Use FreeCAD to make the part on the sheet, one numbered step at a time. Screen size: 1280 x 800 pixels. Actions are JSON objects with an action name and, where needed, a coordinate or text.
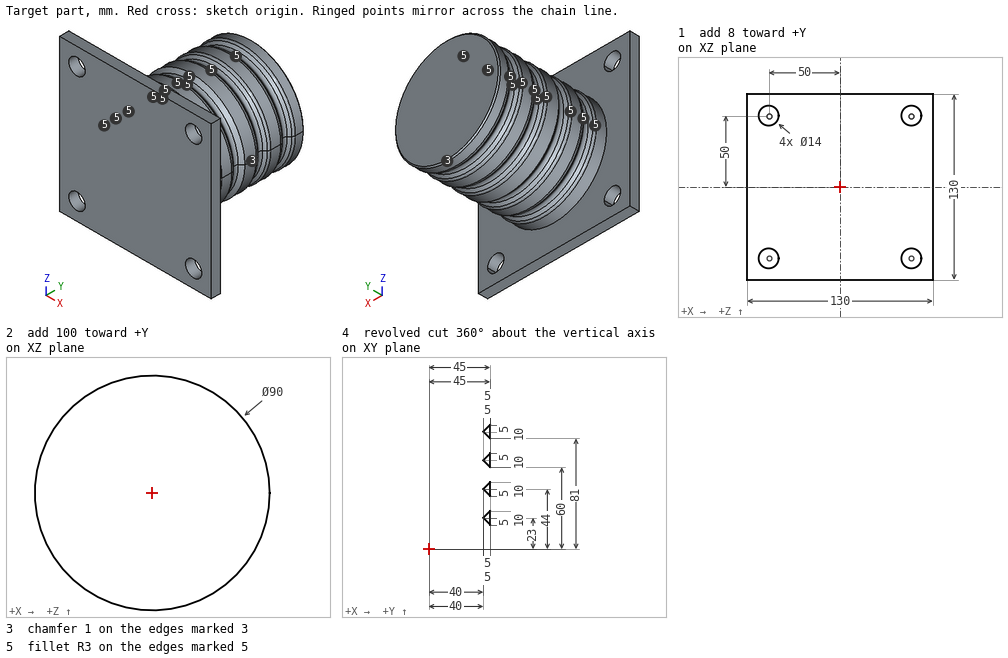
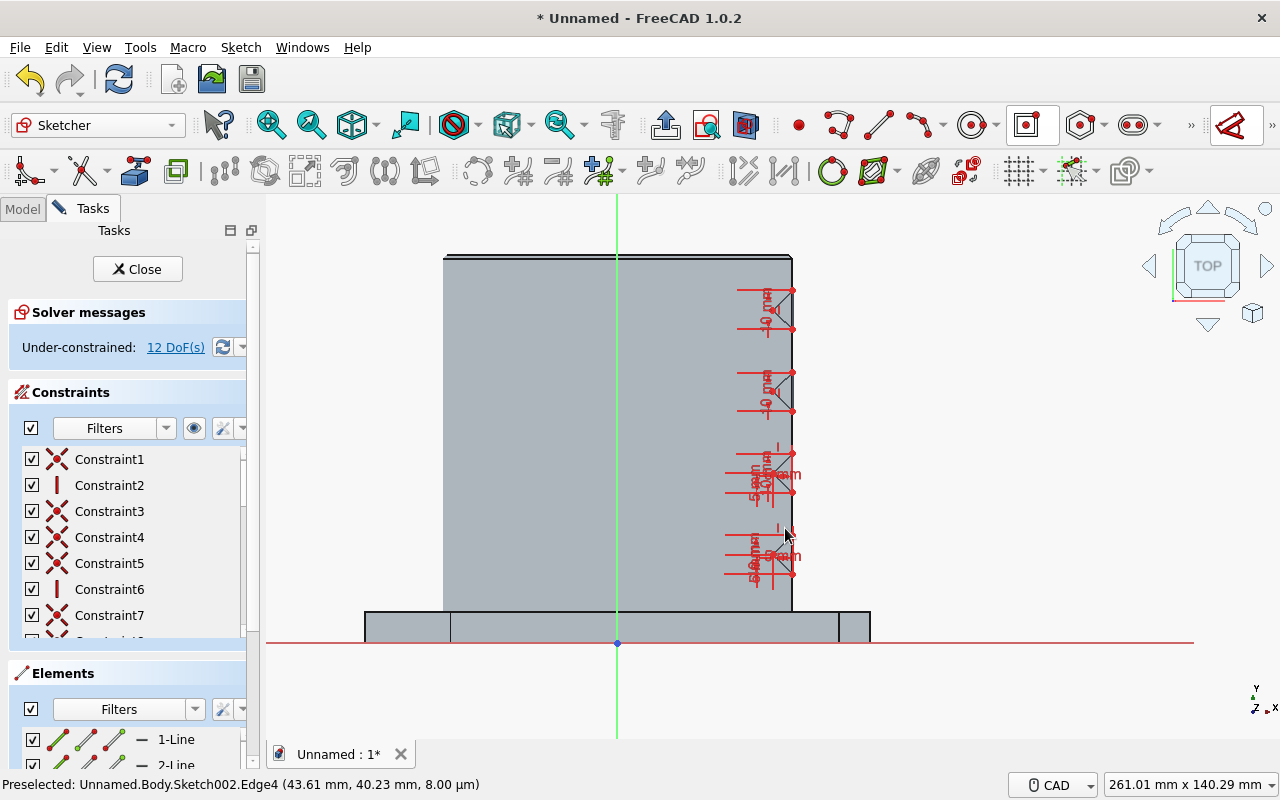
{"action": "scroll", "coordinate": [787, 378], "scroll_direction": "up", "scroll_amount": 5}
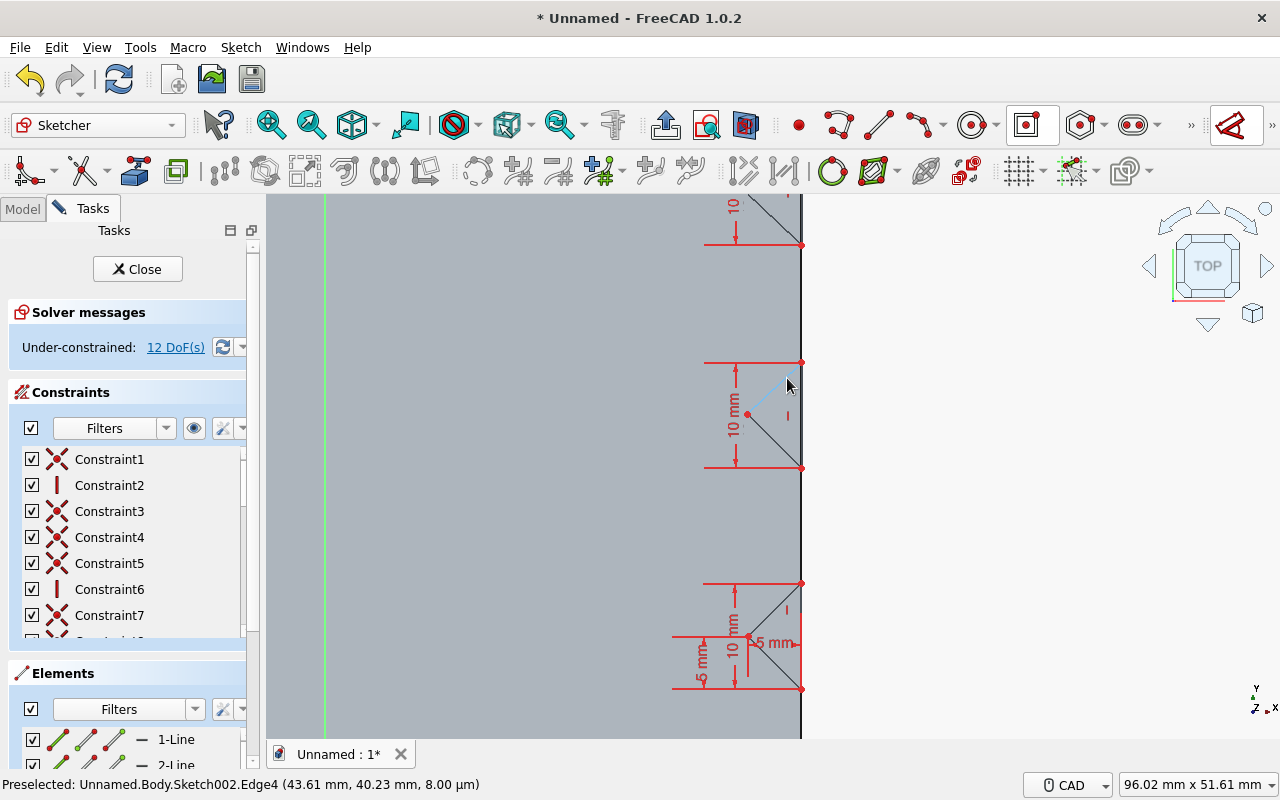
{"action": "left_click", "coordinate": [786, 378]}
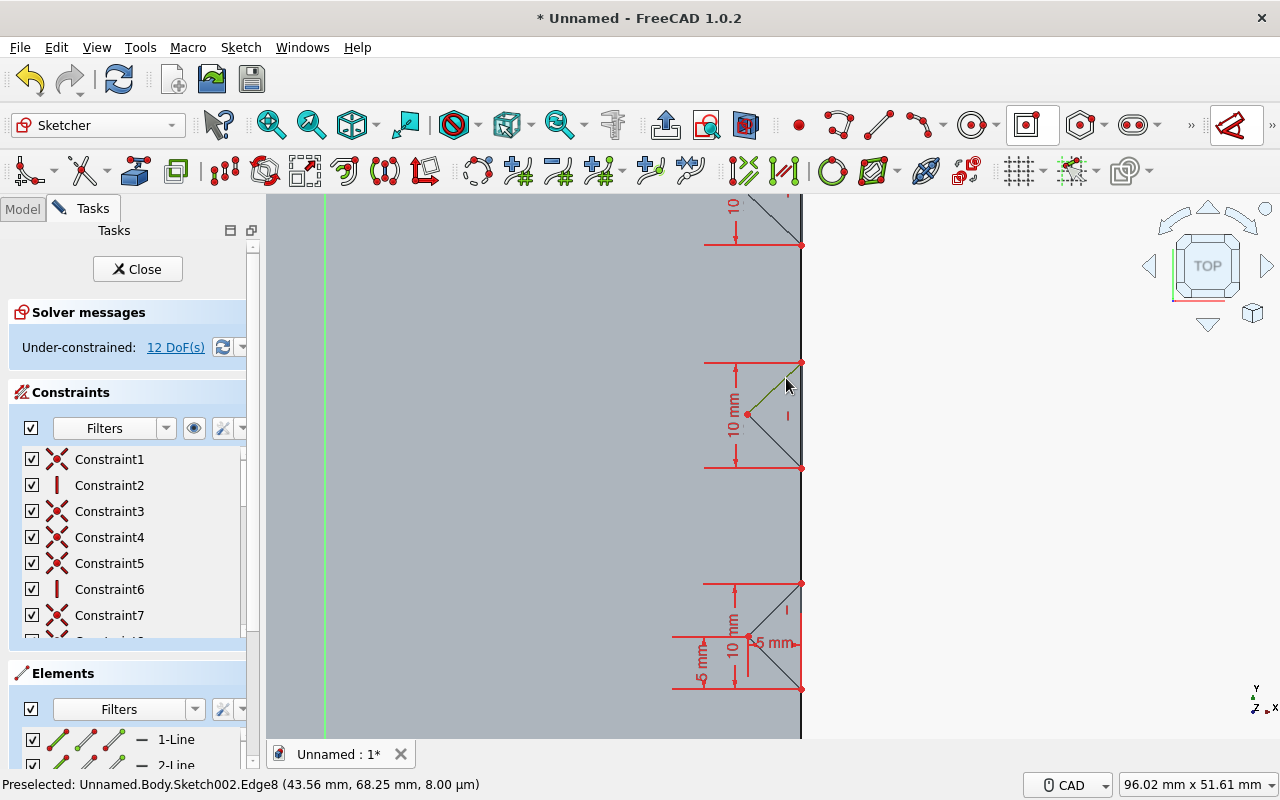
{"action": "left_click", "coordinate": [1258, 126]}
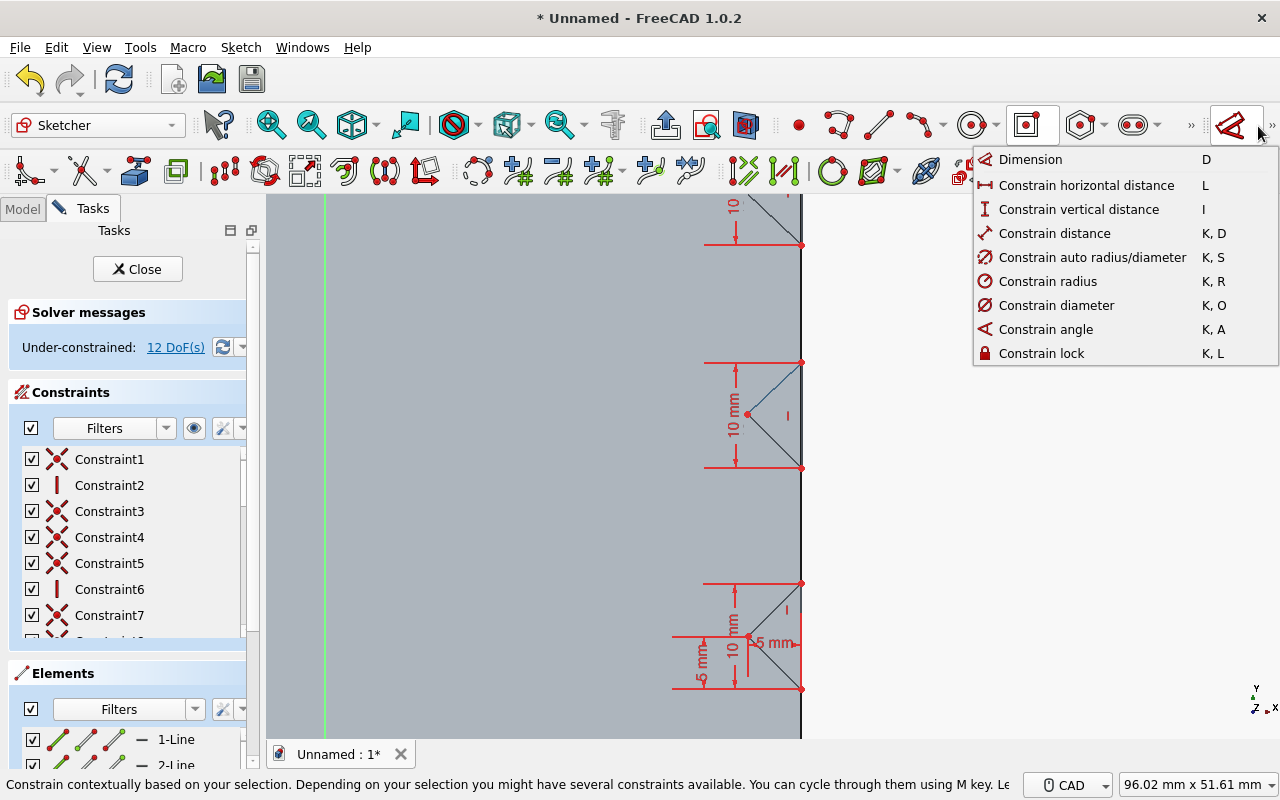
{"action": "left_click", "coordinate": [1126, 185]}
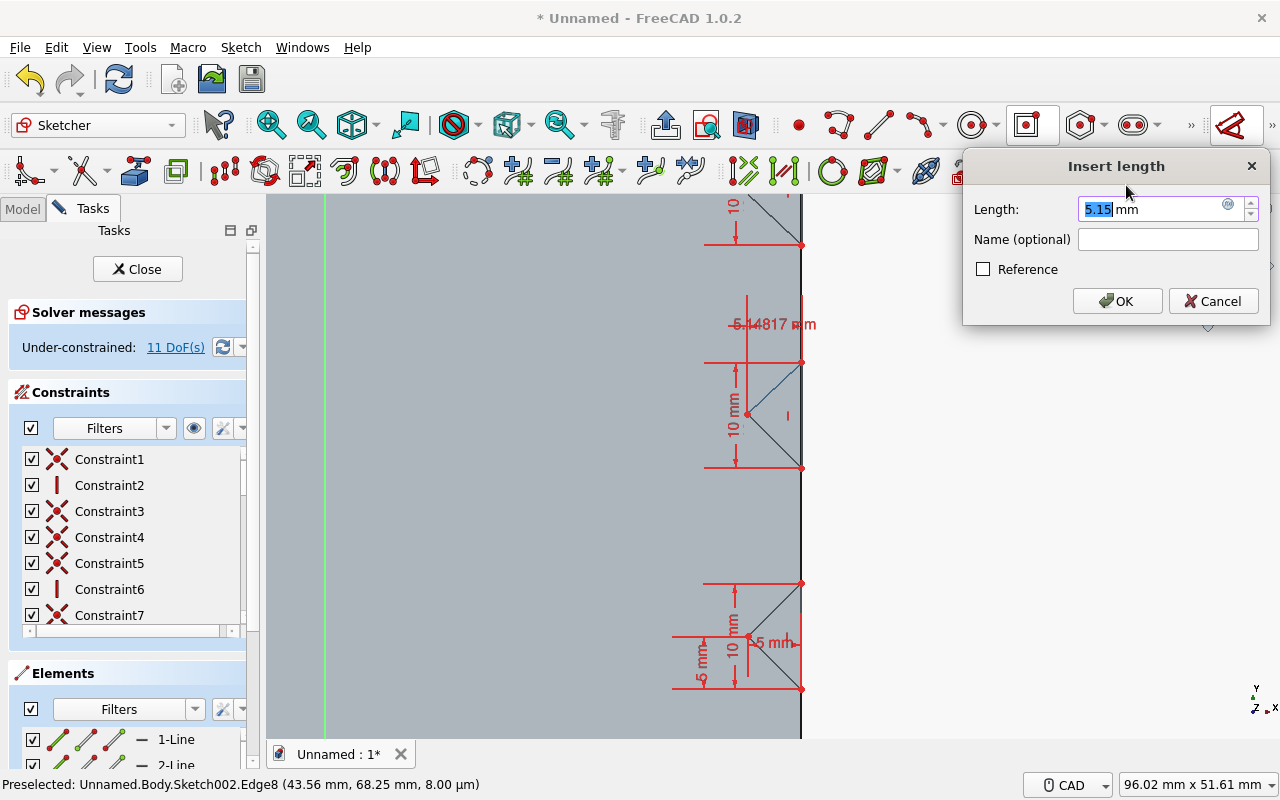
{"action": "type", "text": "5"}
{"action": "key", "text": "Return"}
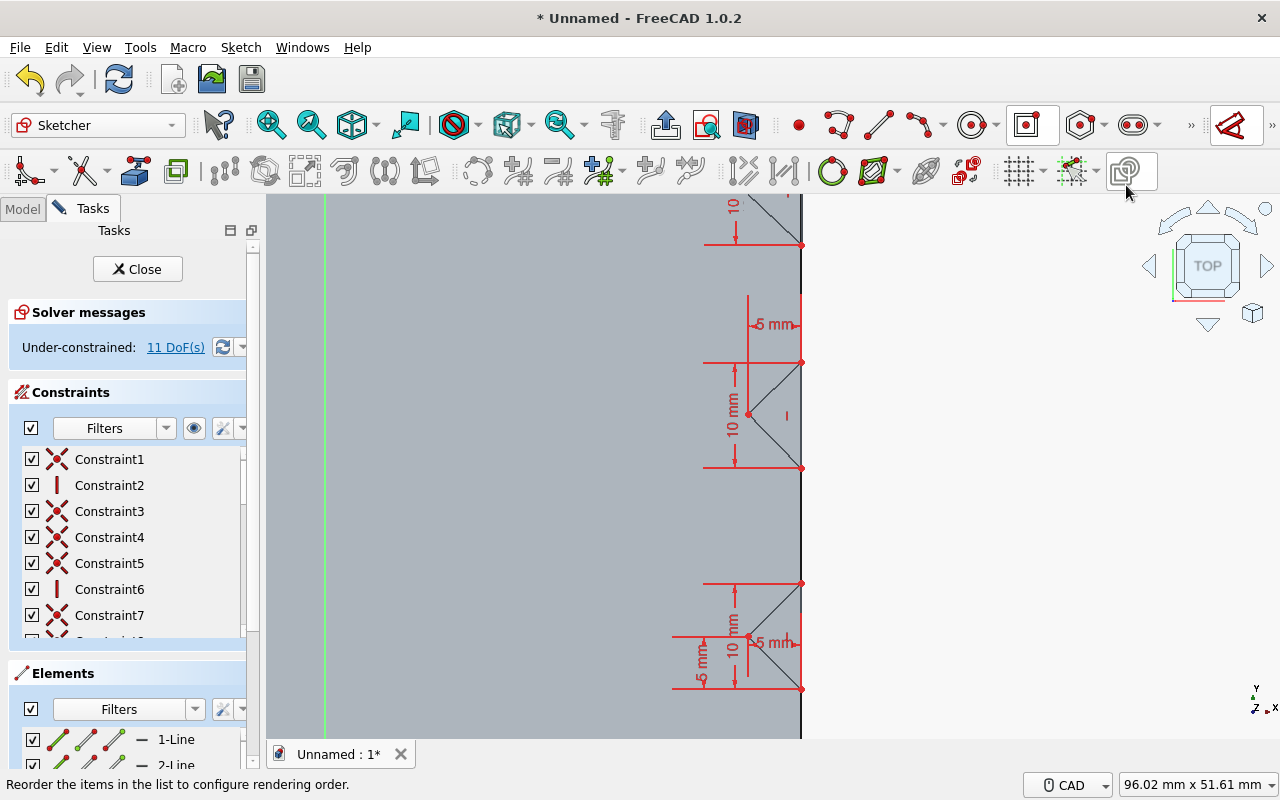
{"action": "left_click", "coordinate": [785, 378]}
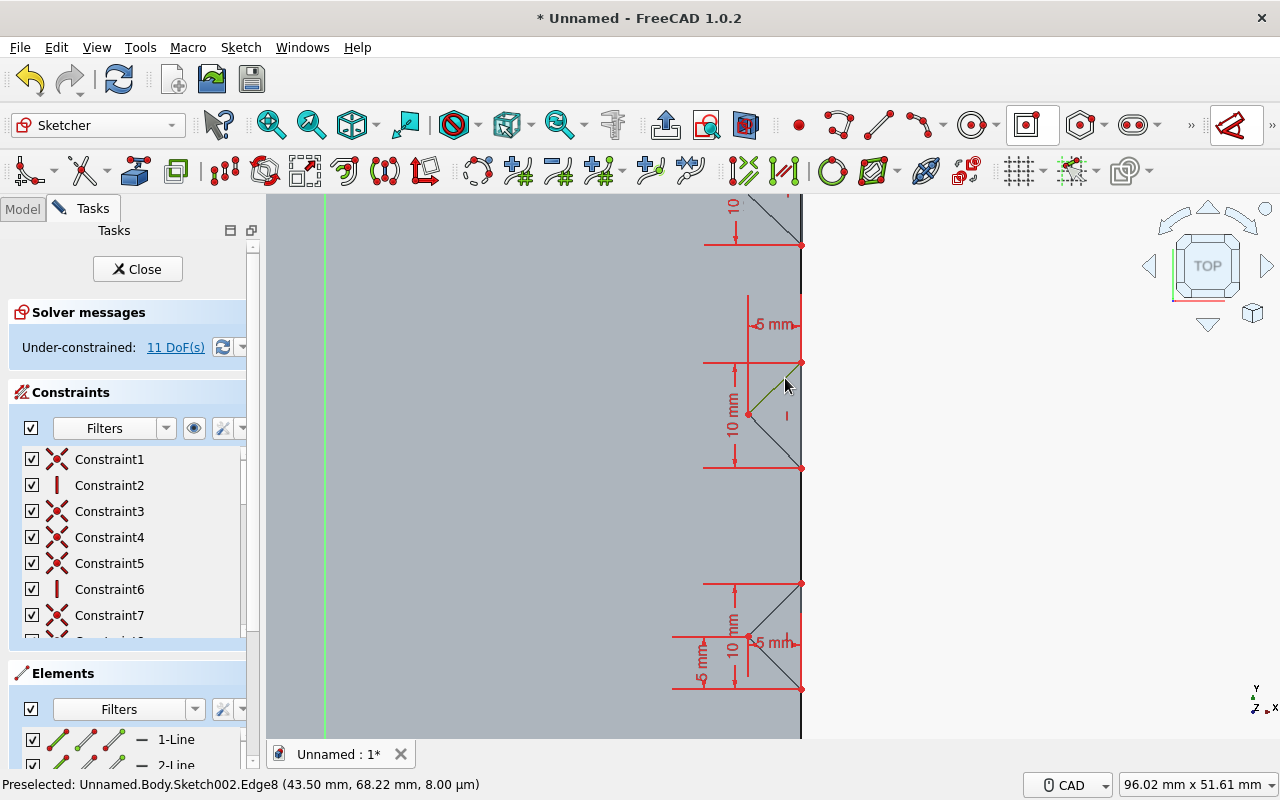
{"action": "left_click", "coordinate": [1258, 126]}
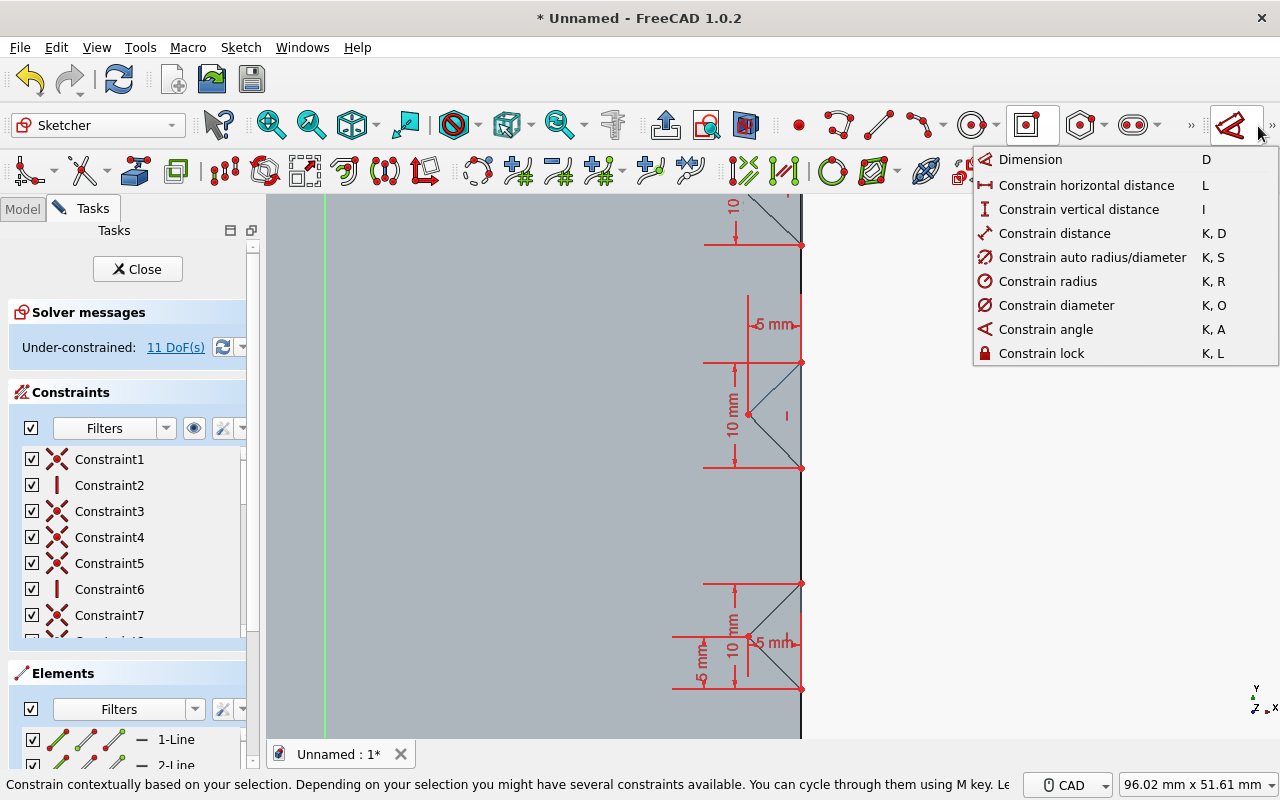
{"action": "left_click", "coordinate": [1126, 209]}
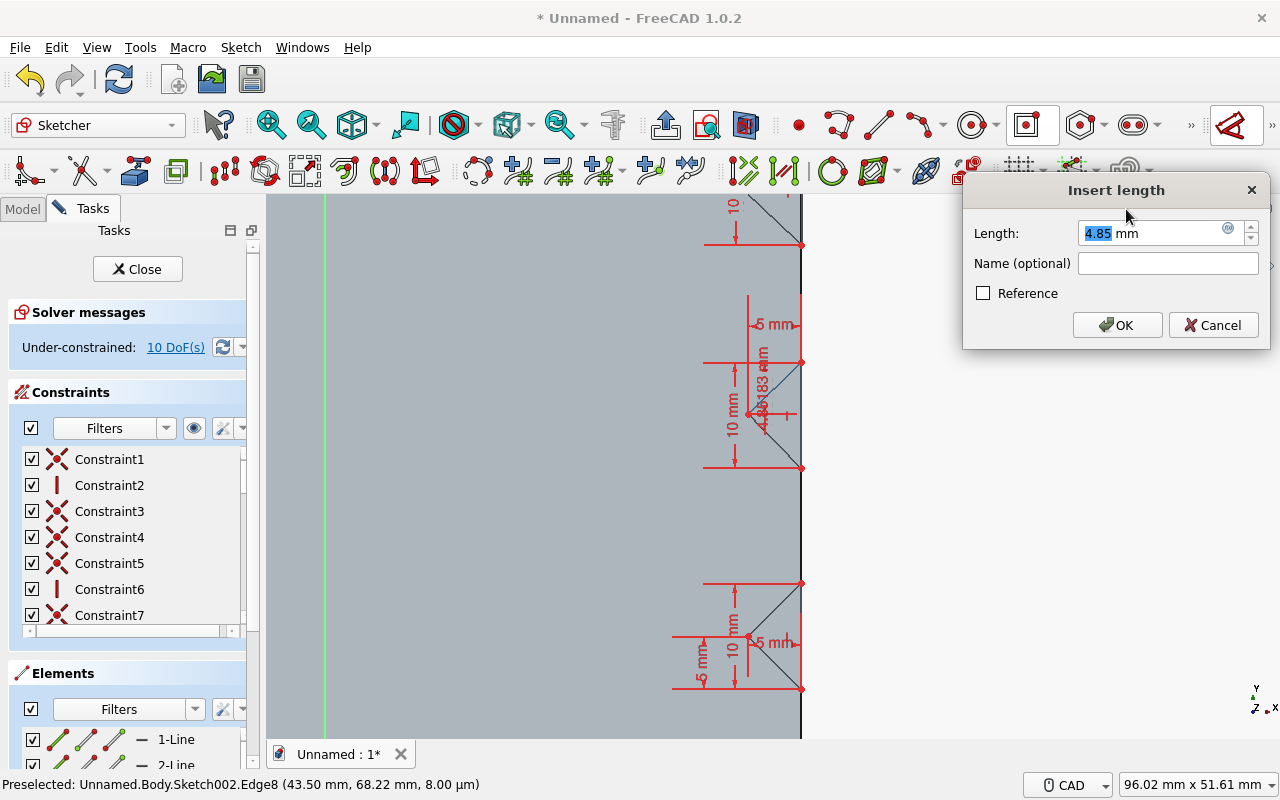
{"action": "type", "text": "5"}
{"action": "key", "text": "Return"}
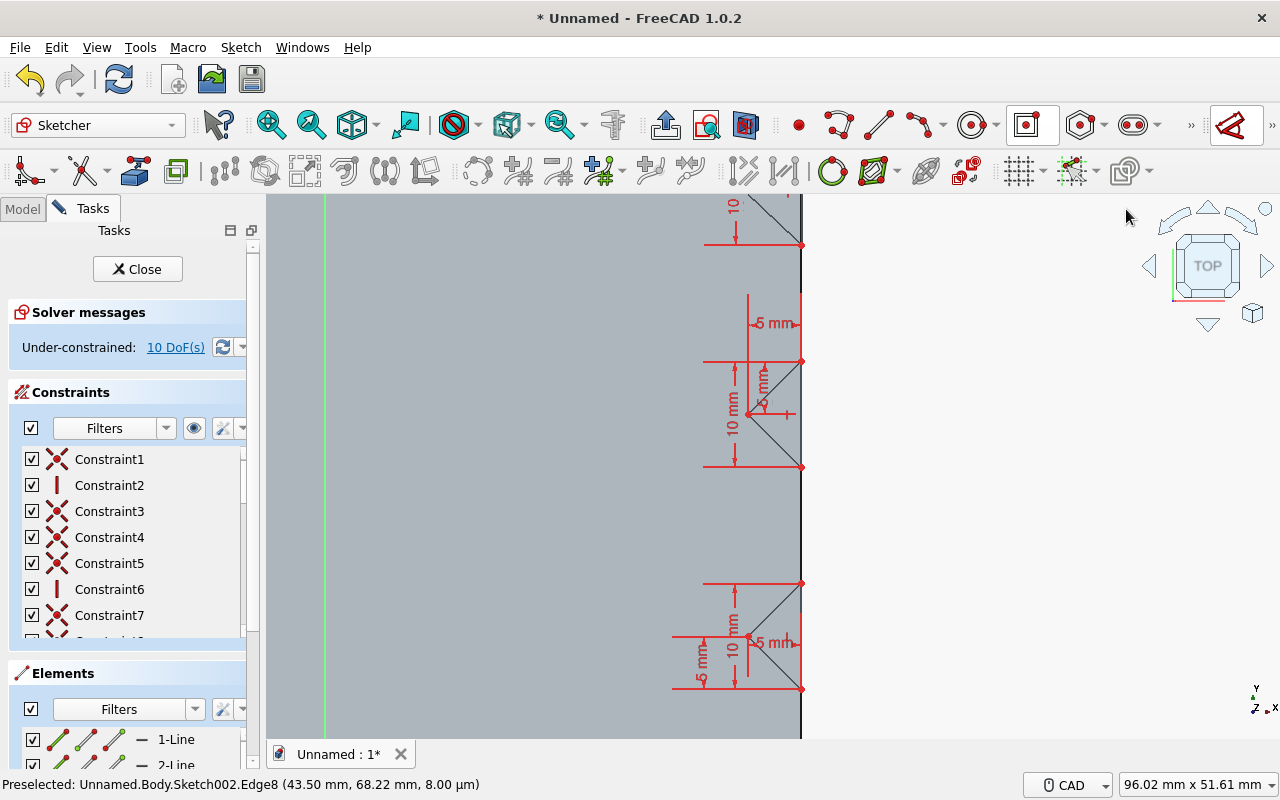
{"action": "scroll", "coordinate": [787, 378], "scroll_direction": "down", "scroll_amount": 5}